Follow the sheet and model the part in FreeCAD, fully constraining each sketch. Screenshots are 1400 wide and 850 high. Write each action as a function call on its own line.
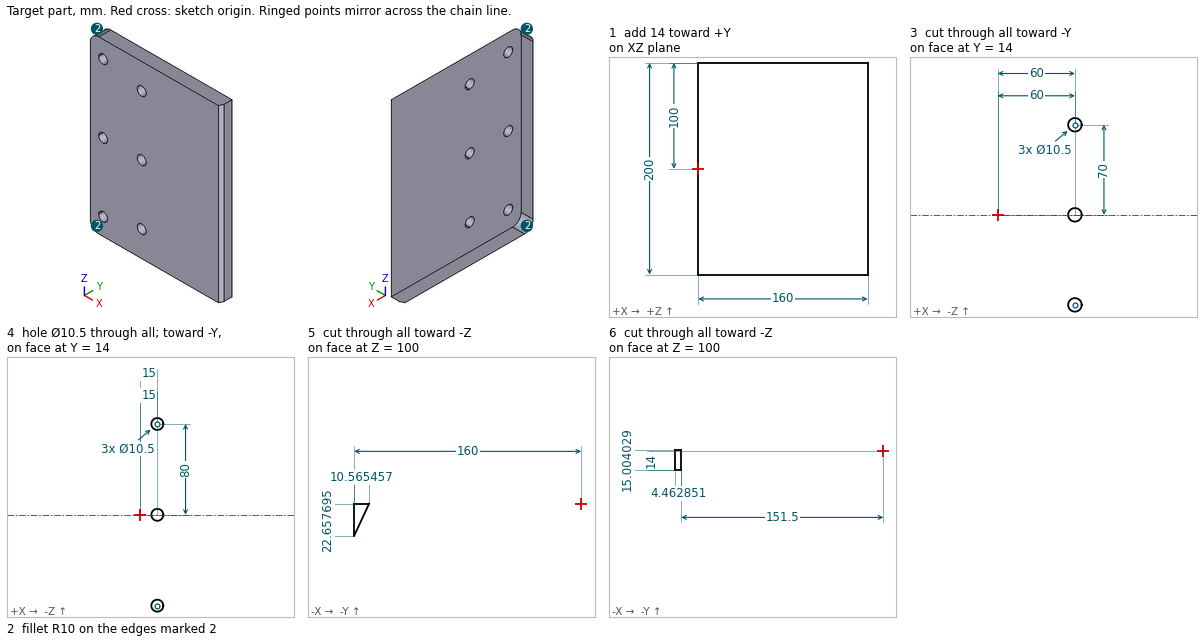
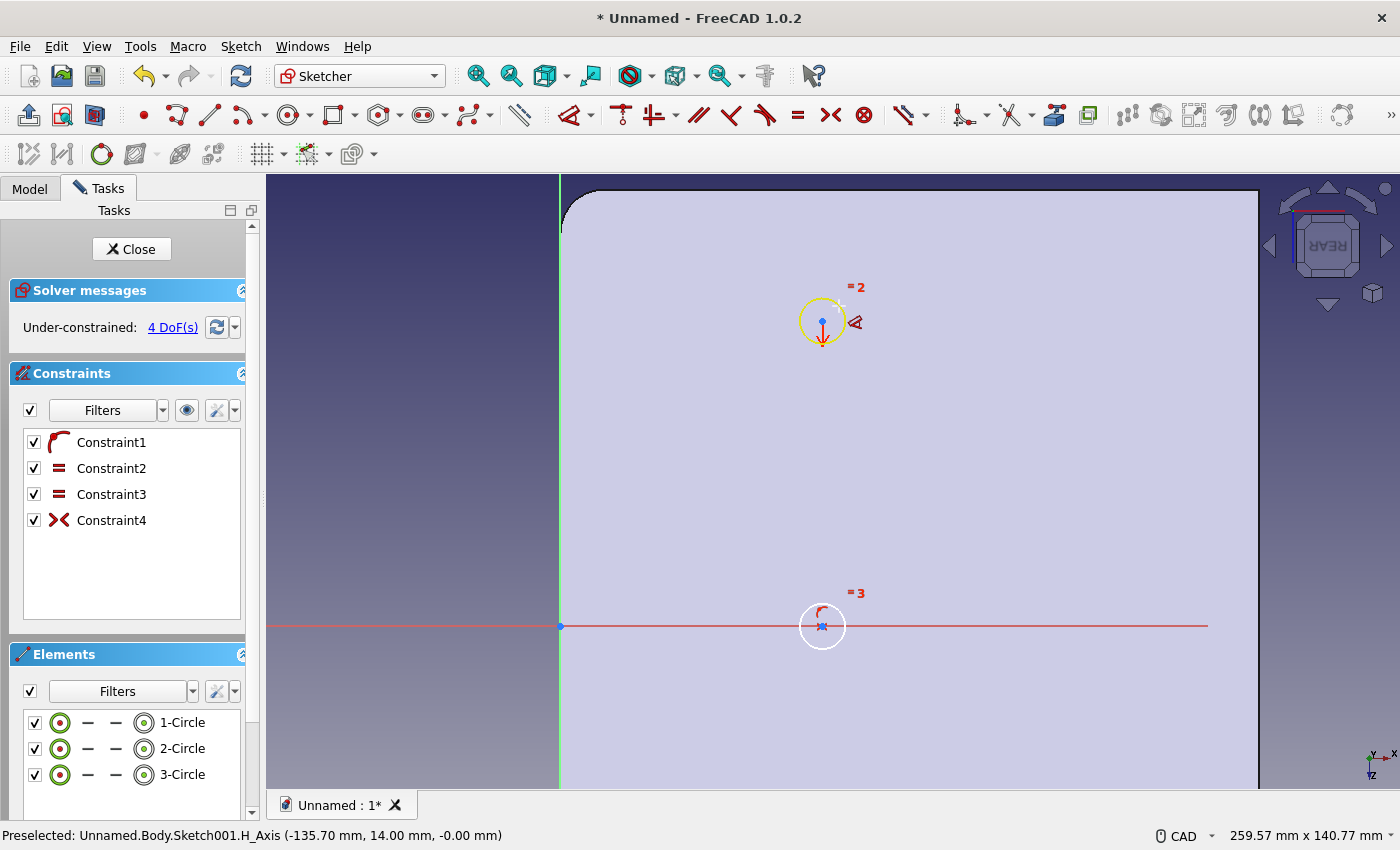
click(839, 305)
click(862, 283)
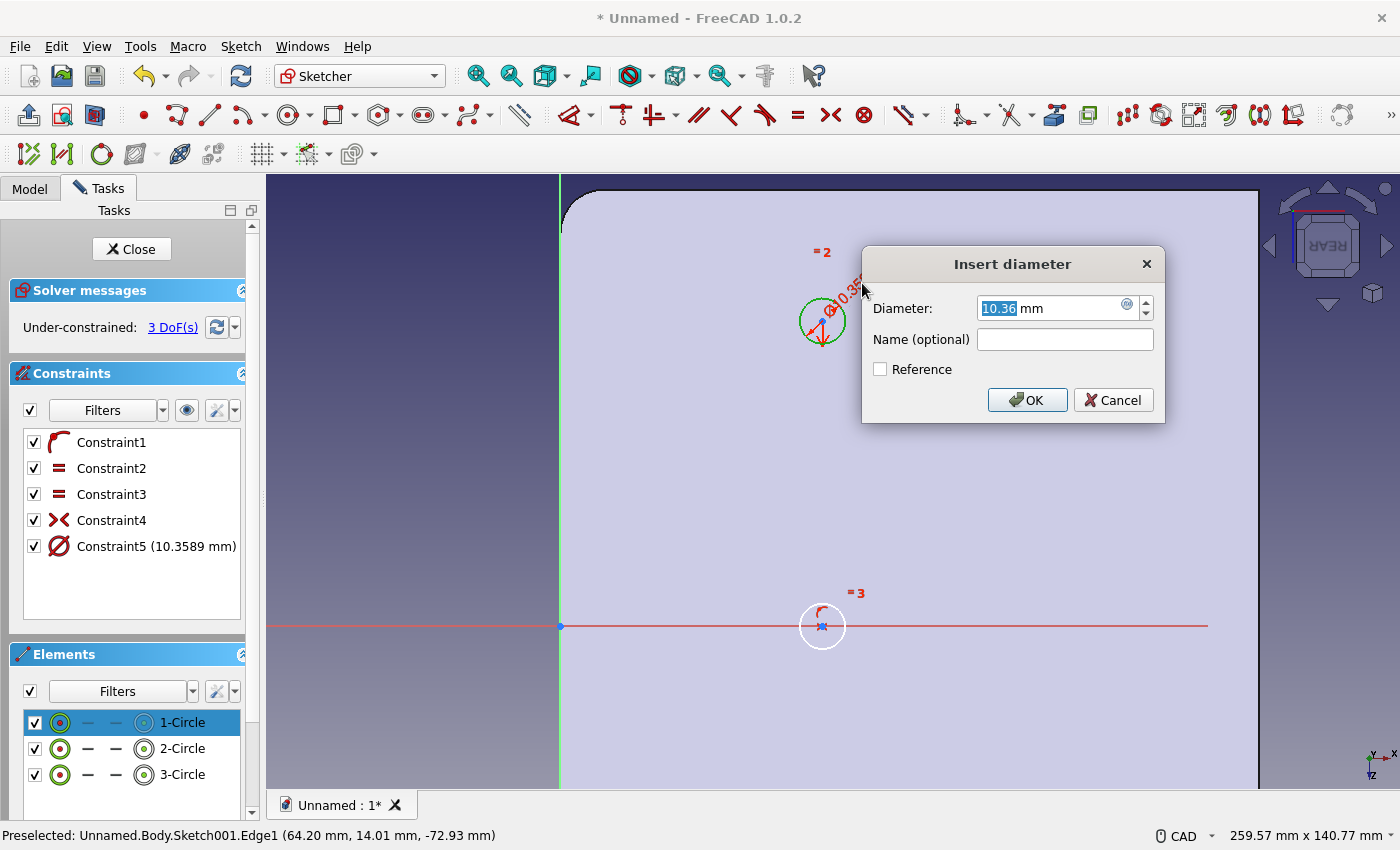
text(10.5)
key(Return)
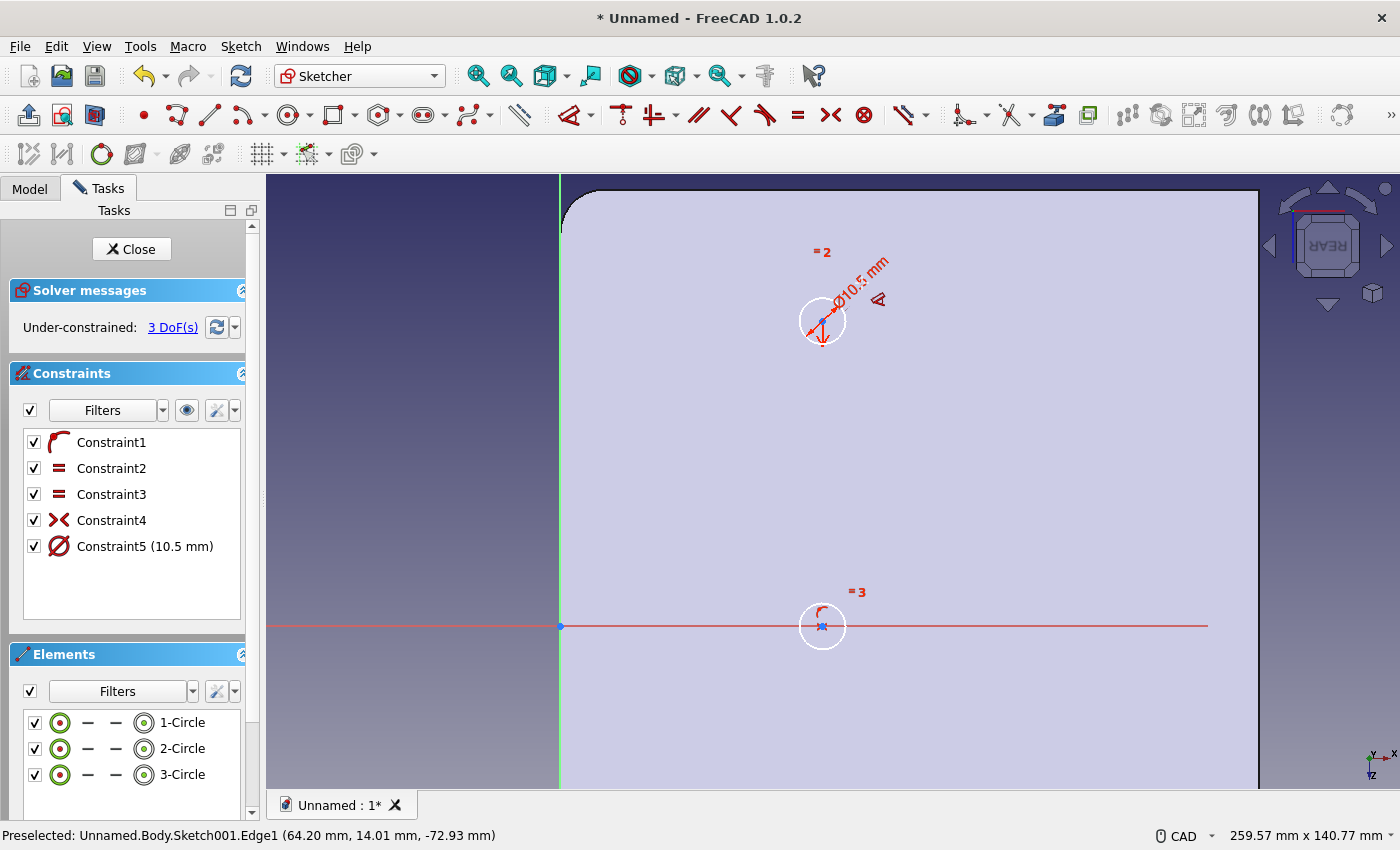
click(823, 321)
click(692, 287)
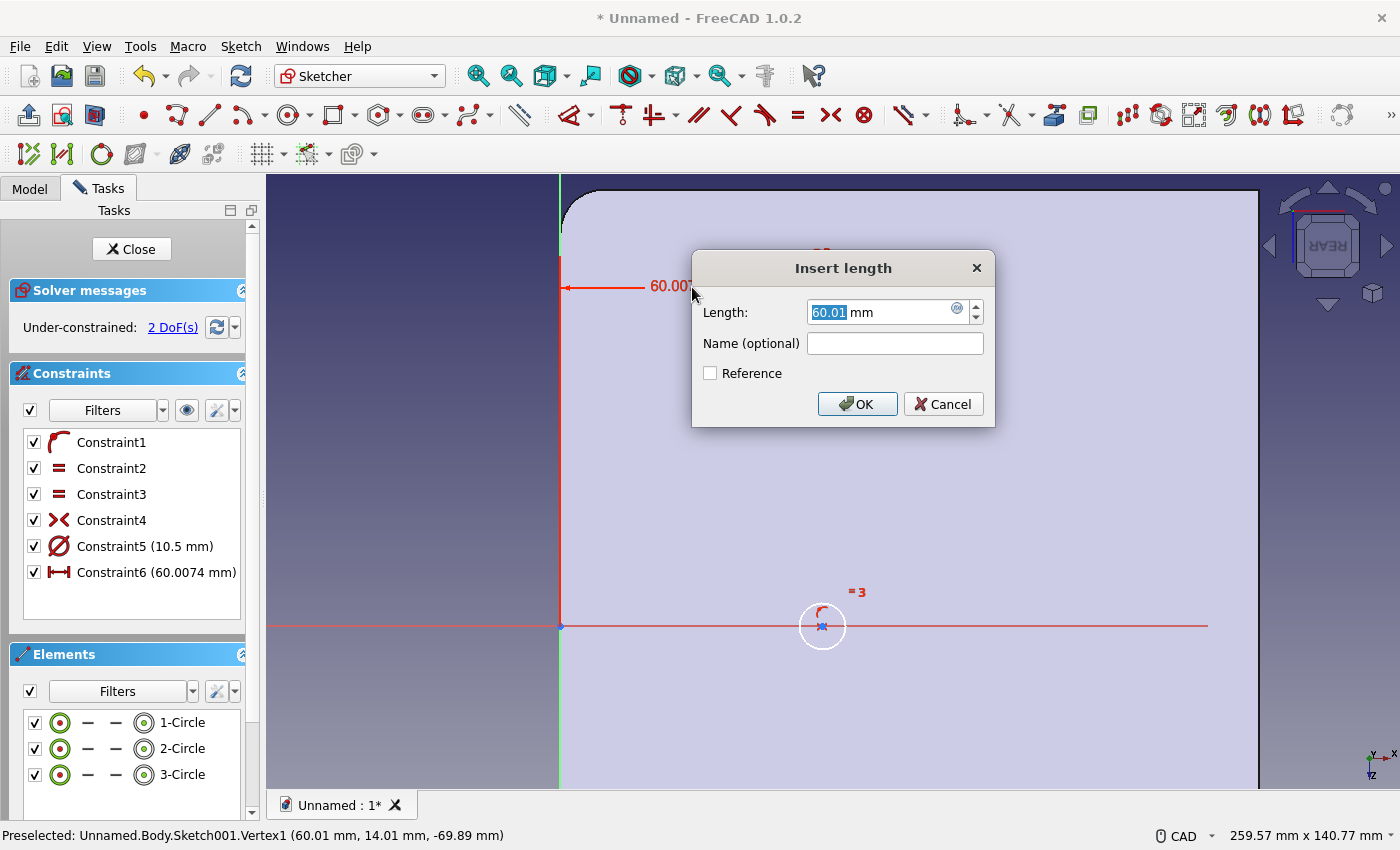
text(60)
key(Return)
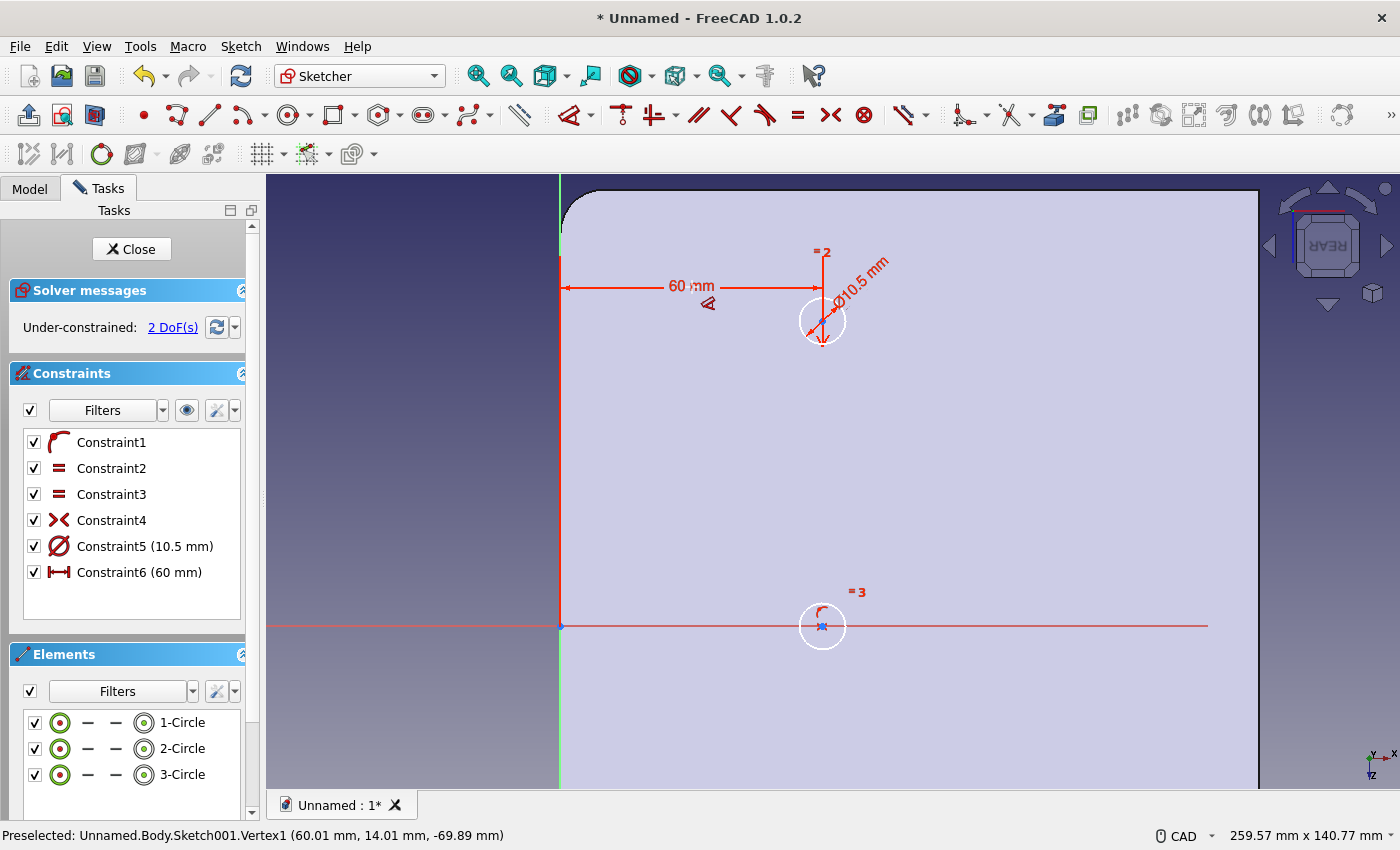
click(823, 321)
click(526, 474)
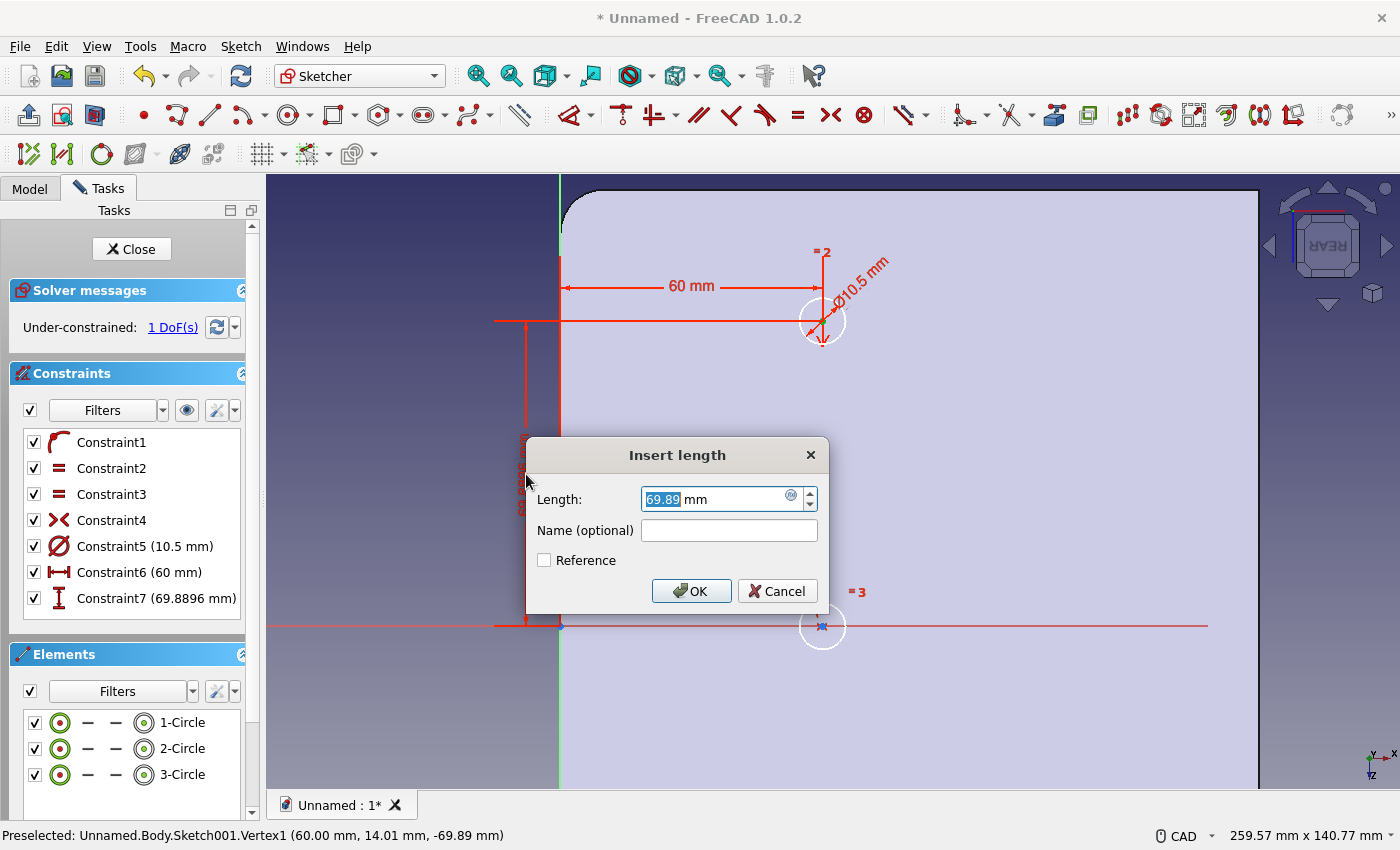
text(70)
key(Return)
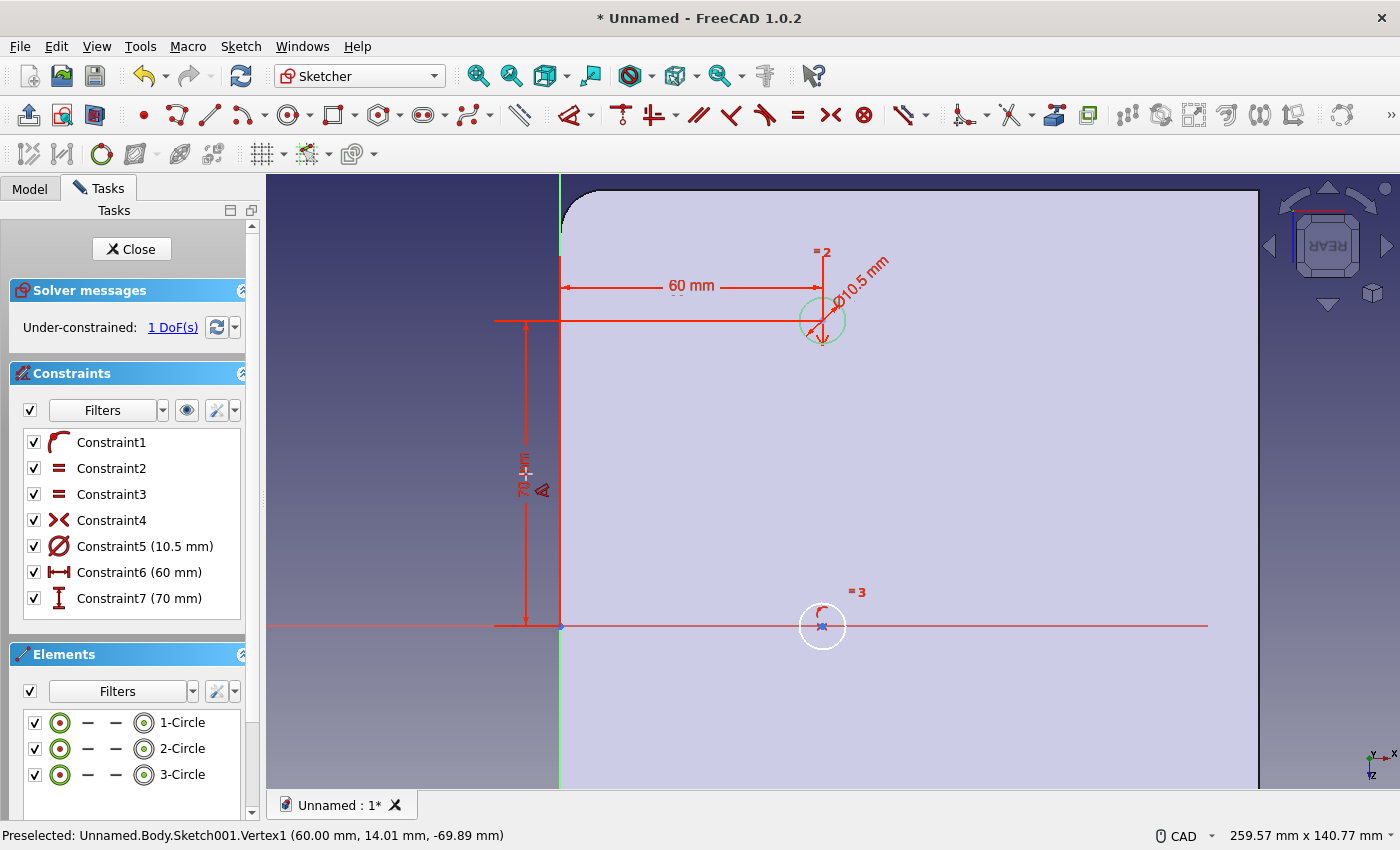
click(823, 626)
click(692, 660)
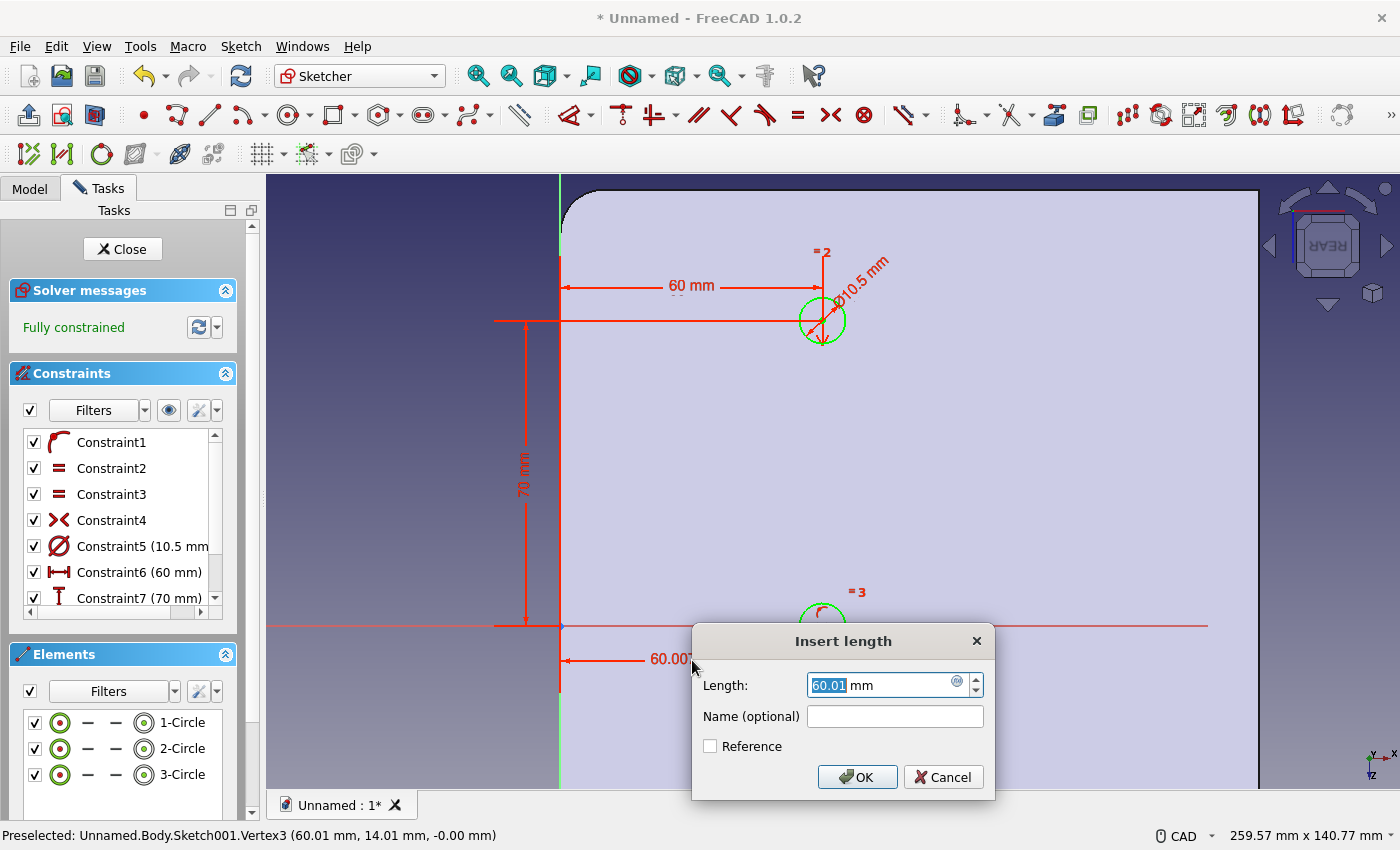
text(60)
key(Return)
key(Escape)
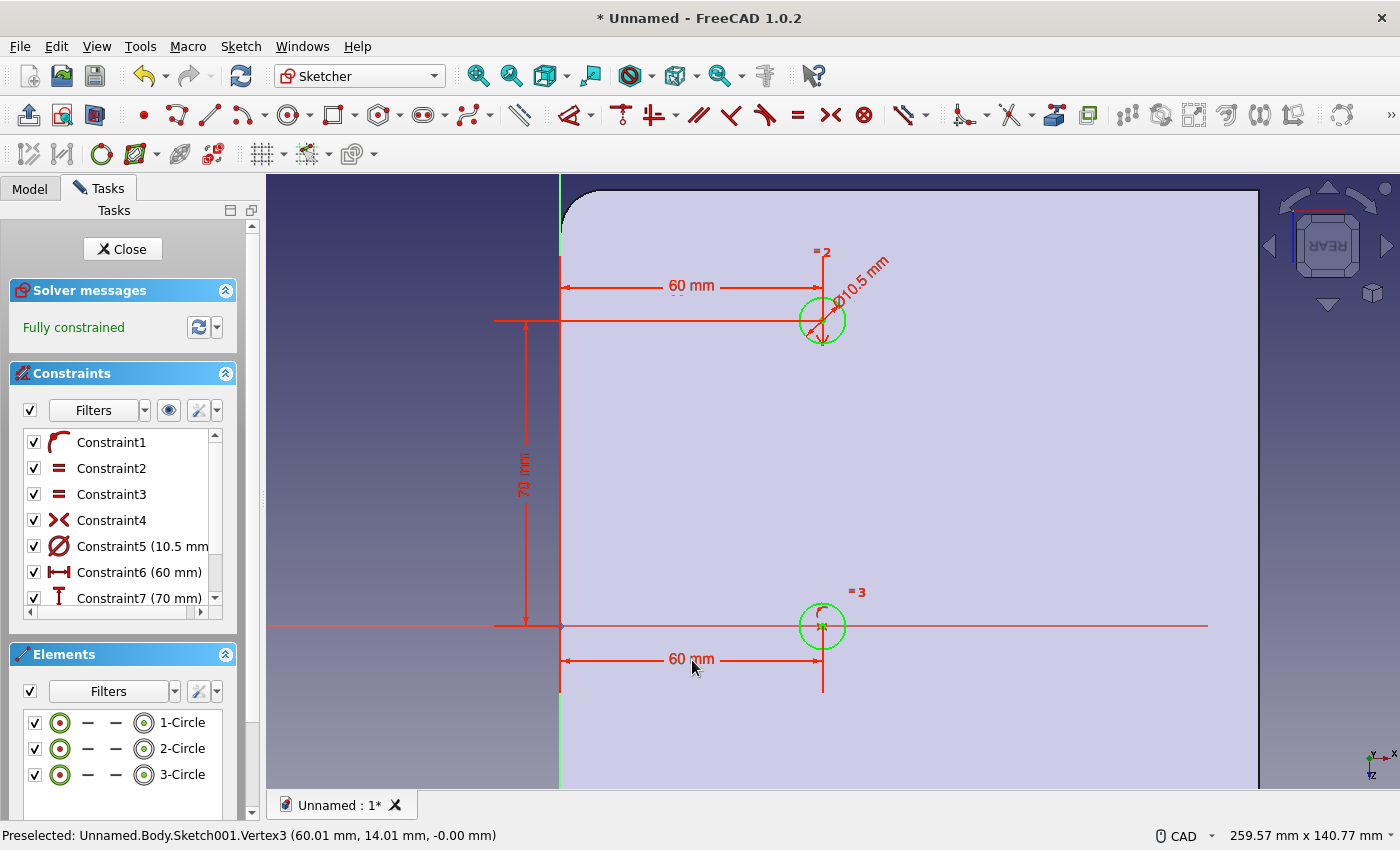
click(123, 249)